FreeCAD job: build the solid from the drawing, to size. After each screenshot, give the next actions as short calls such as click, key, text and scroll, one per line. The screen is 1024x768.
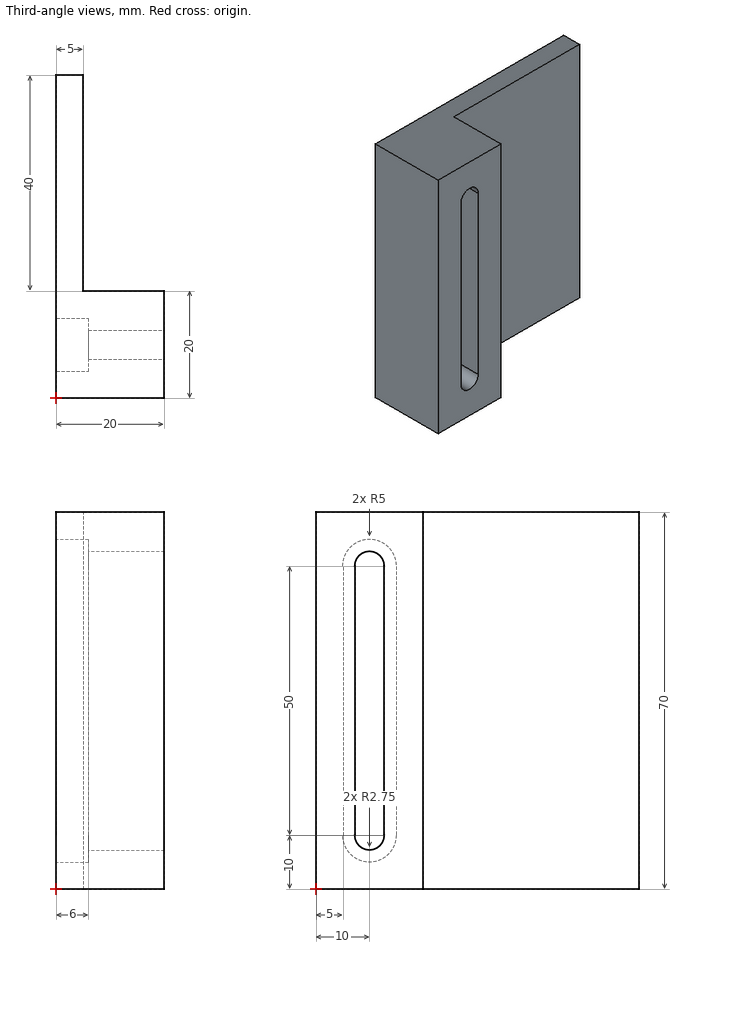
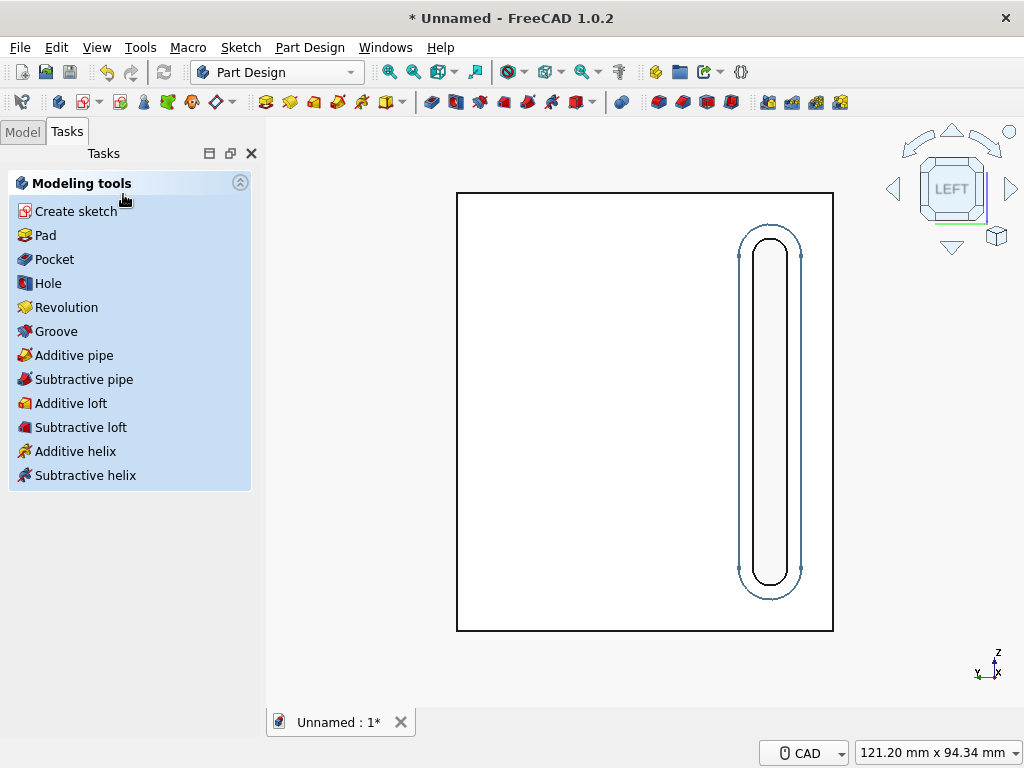
click(432, 102)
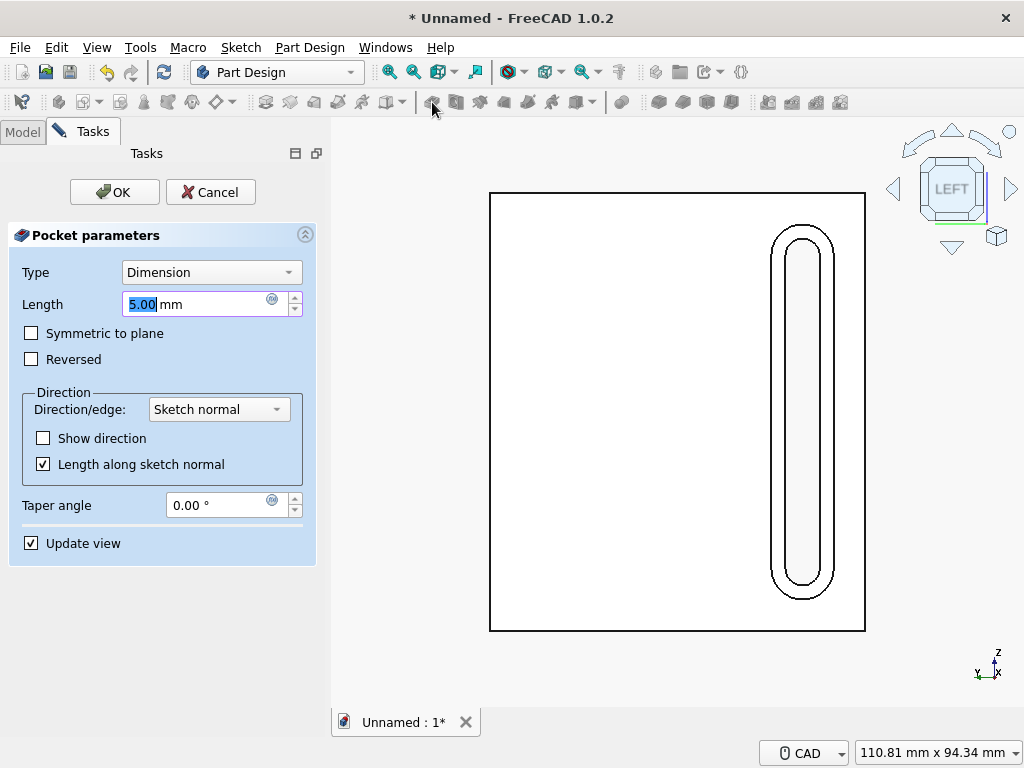
text(6)
key(Tab)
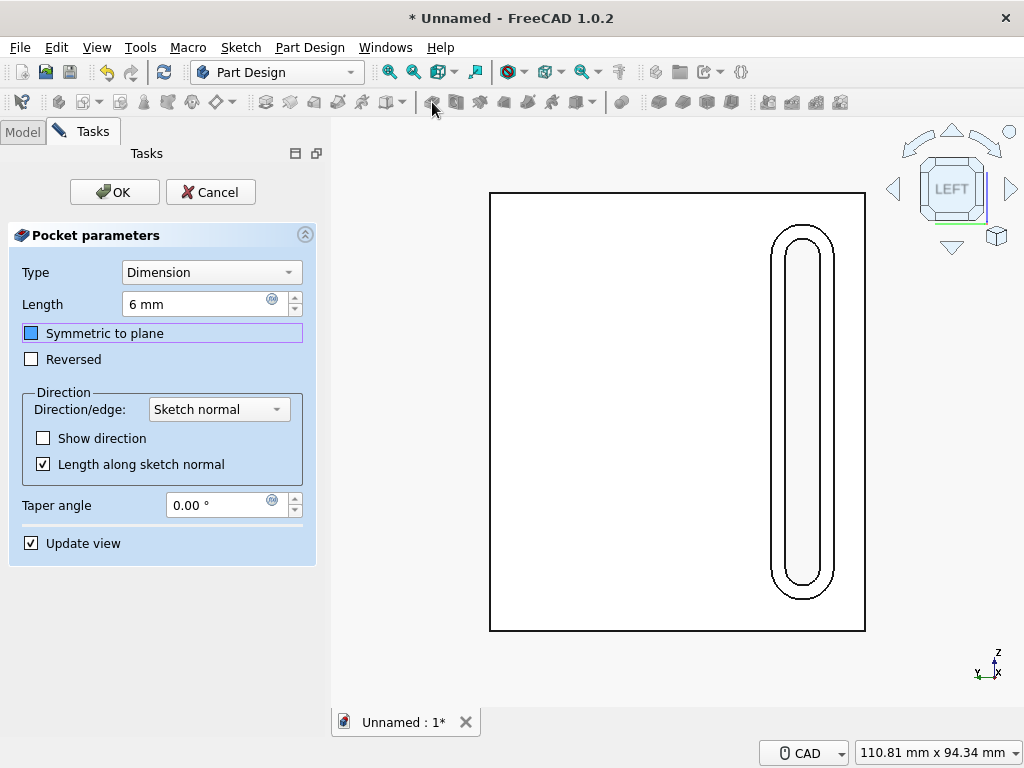
click(115, 192)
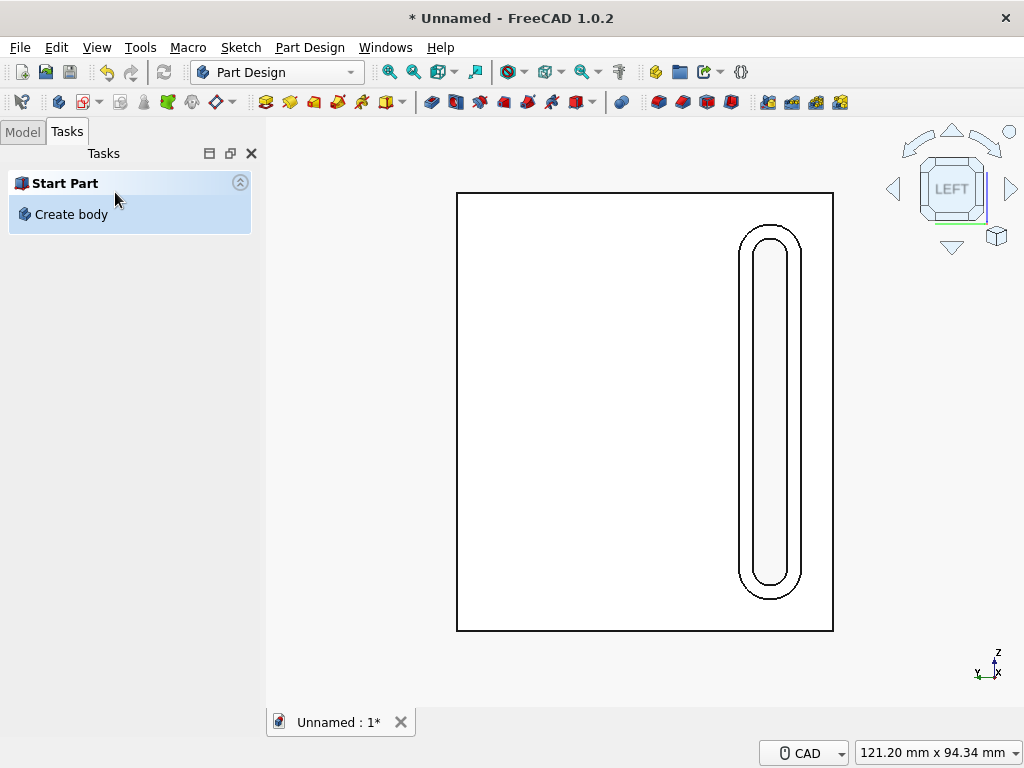
key(0)